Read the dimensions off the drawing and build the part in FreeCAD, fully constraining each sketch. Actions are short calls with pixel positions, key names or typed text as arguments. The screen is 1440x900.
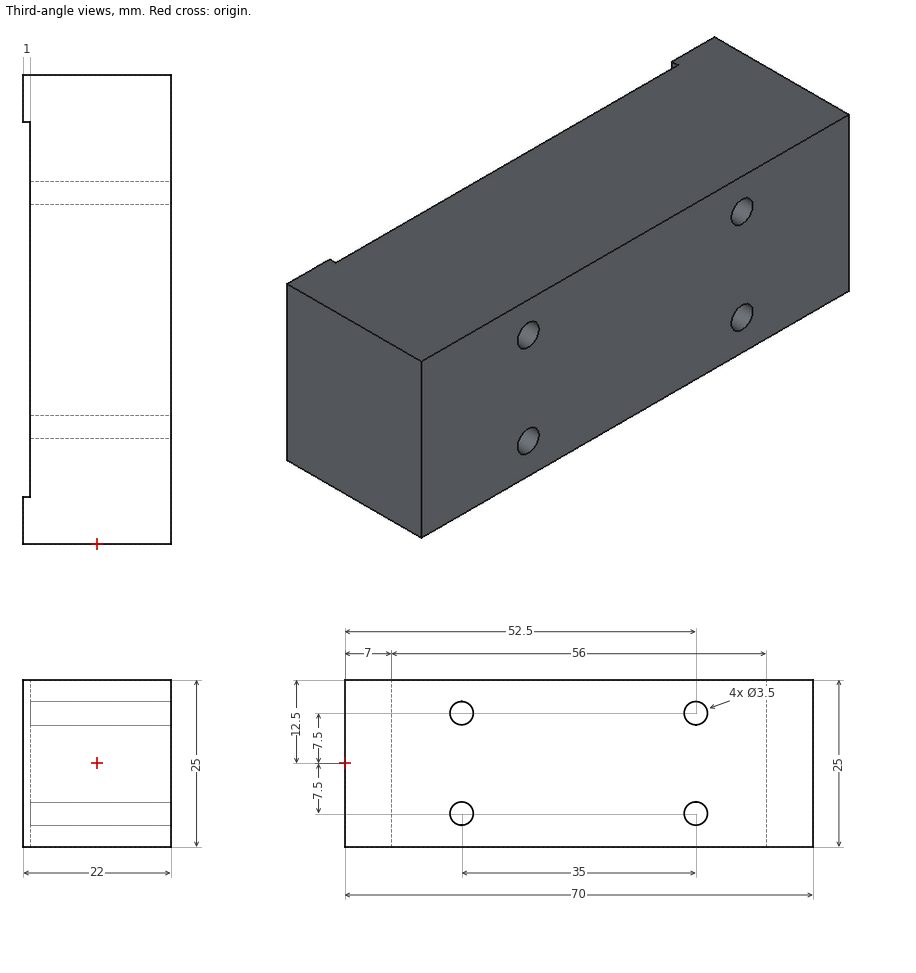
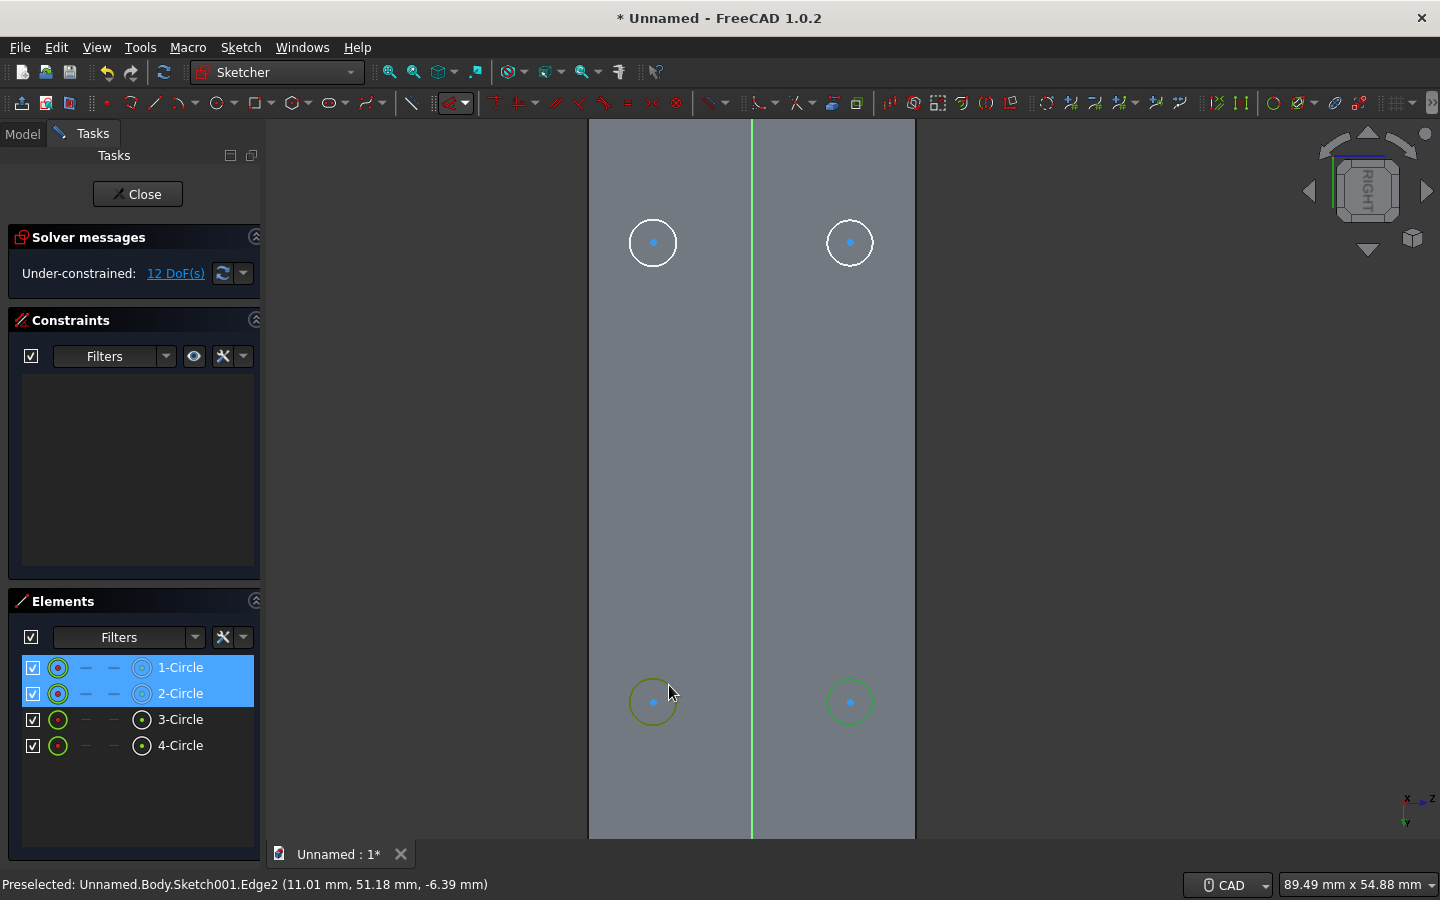
click(669, 226)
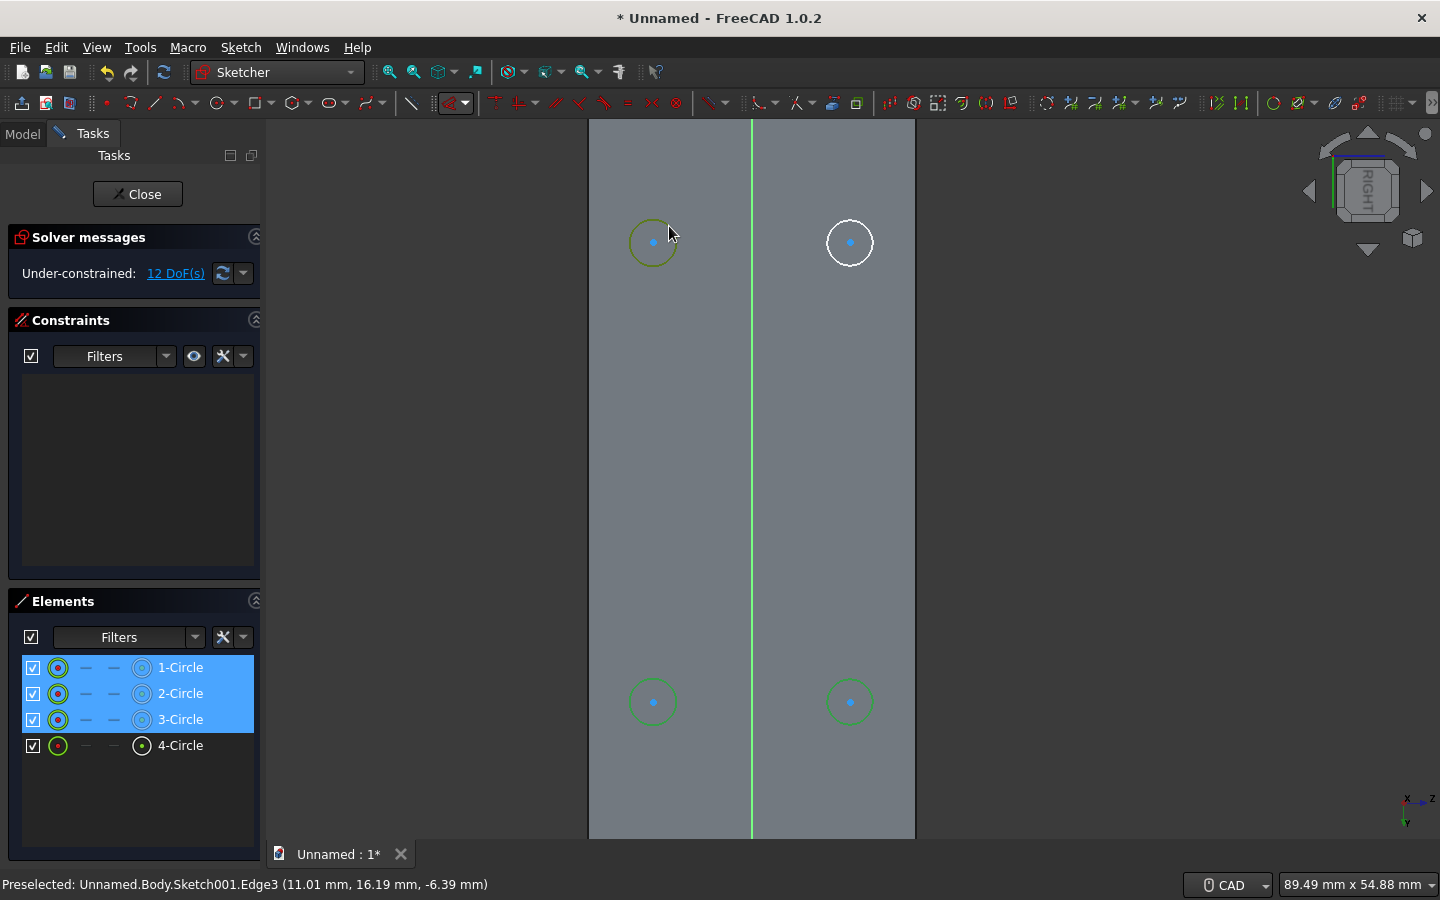
click(866, 227)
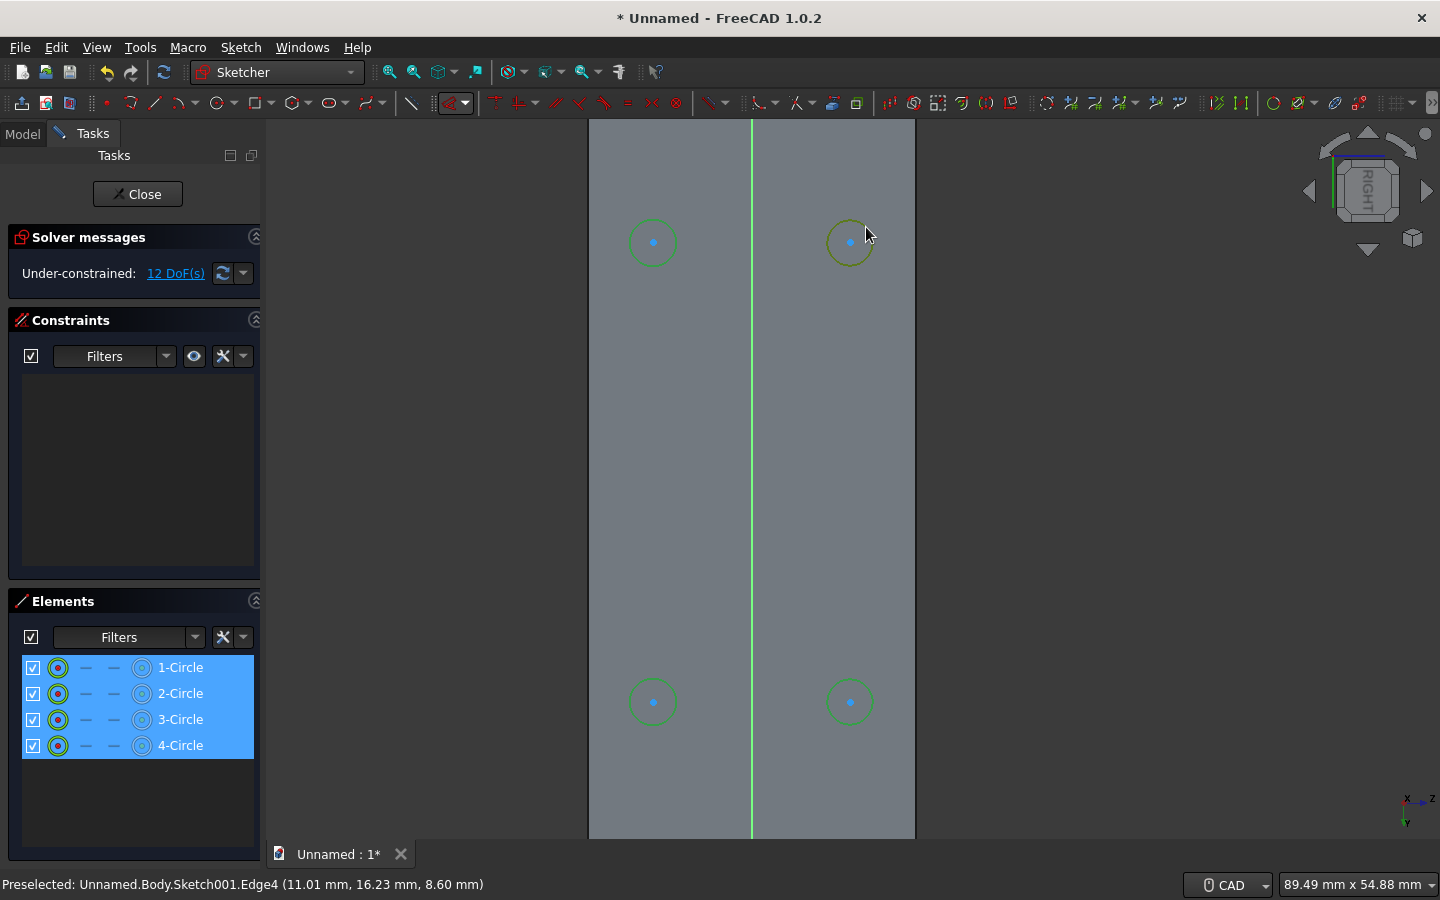
click(628, 104)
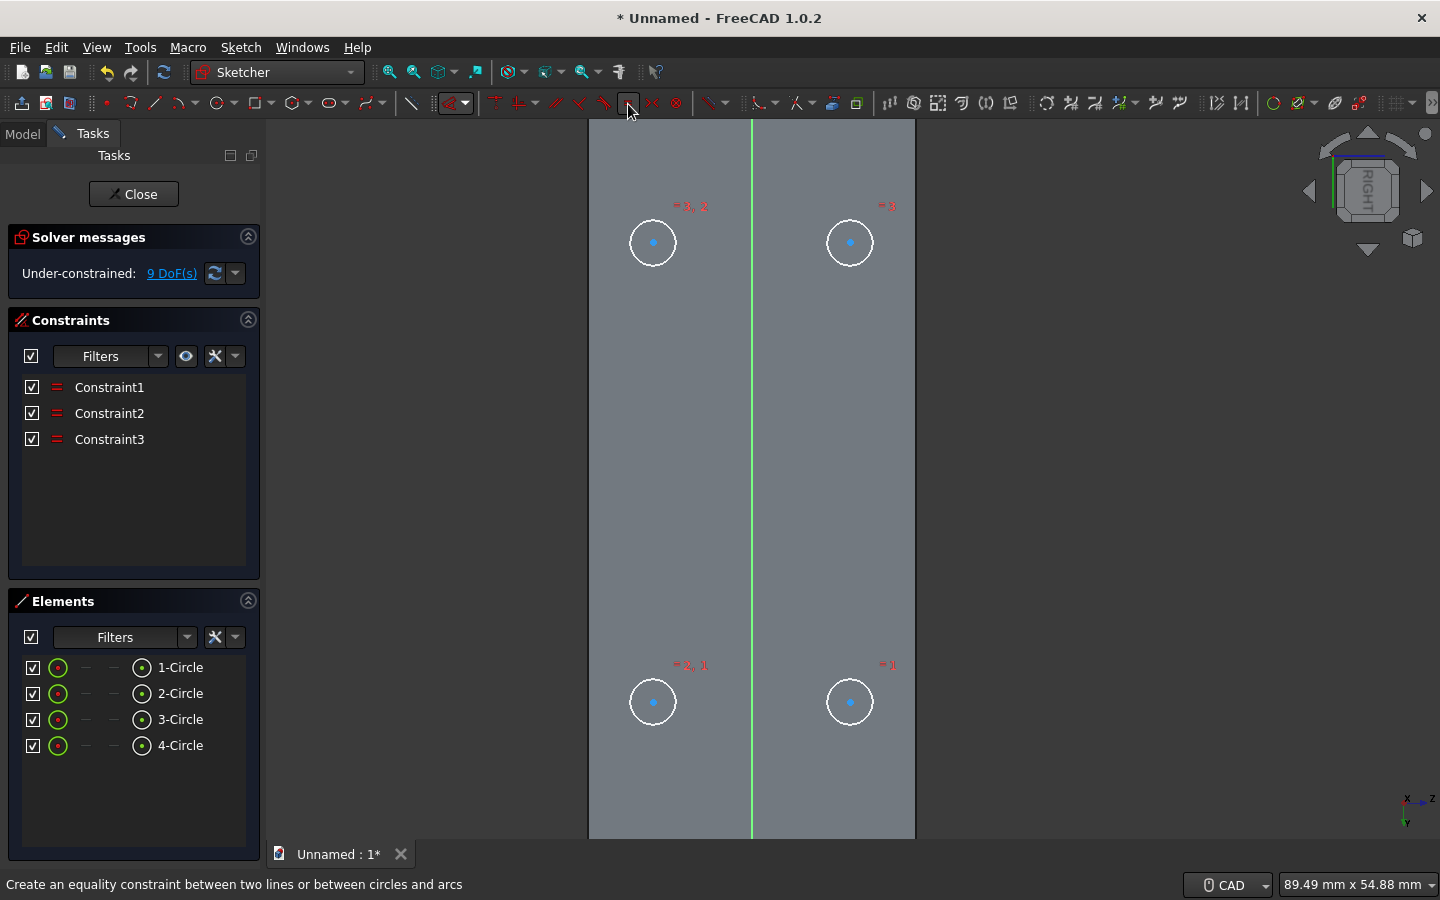
click(850, 702)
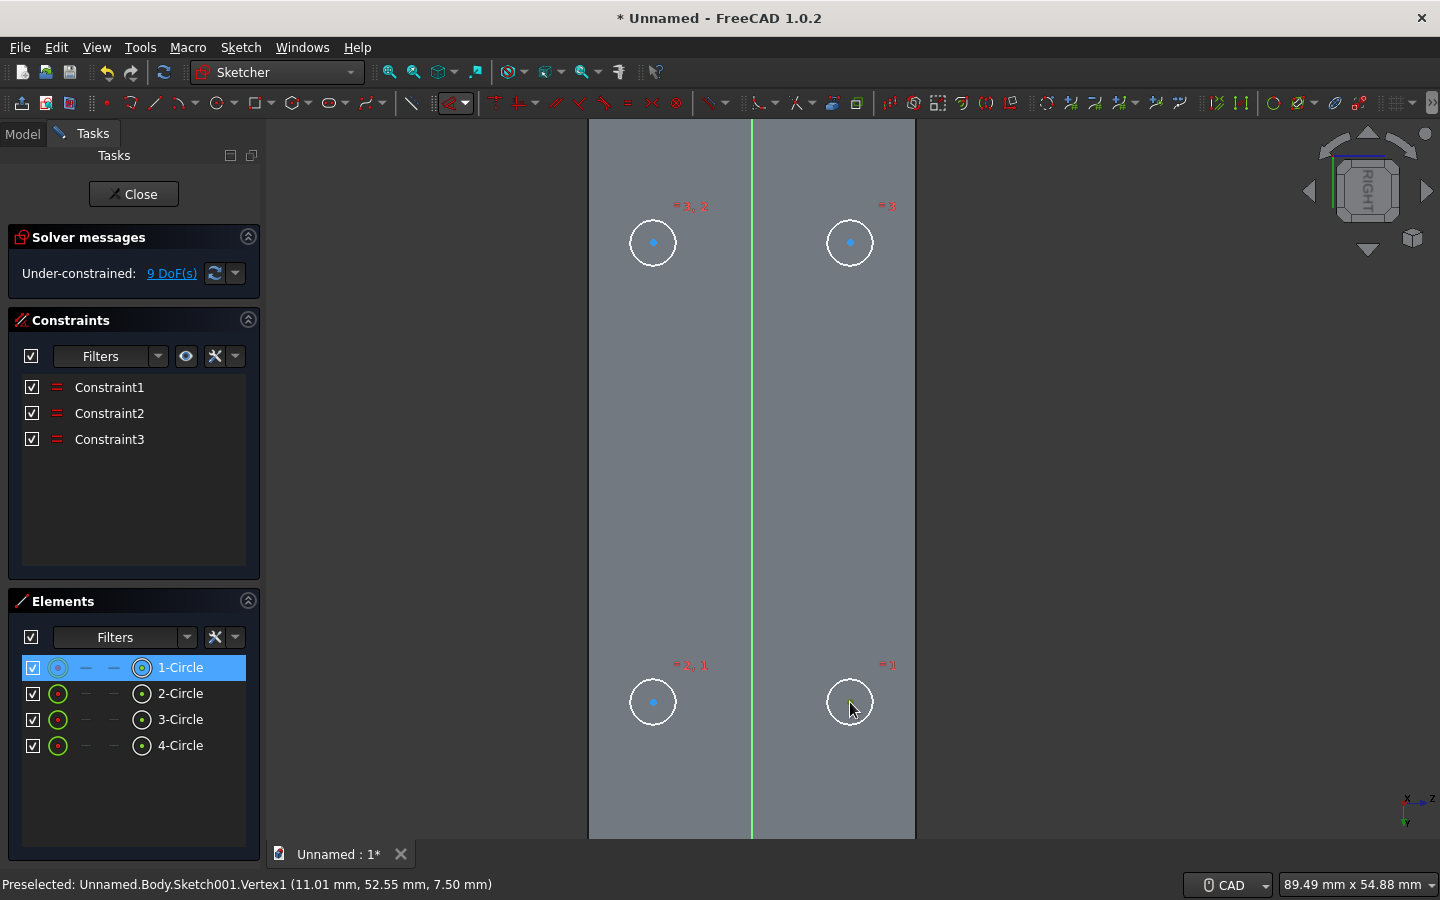
click(653, 702)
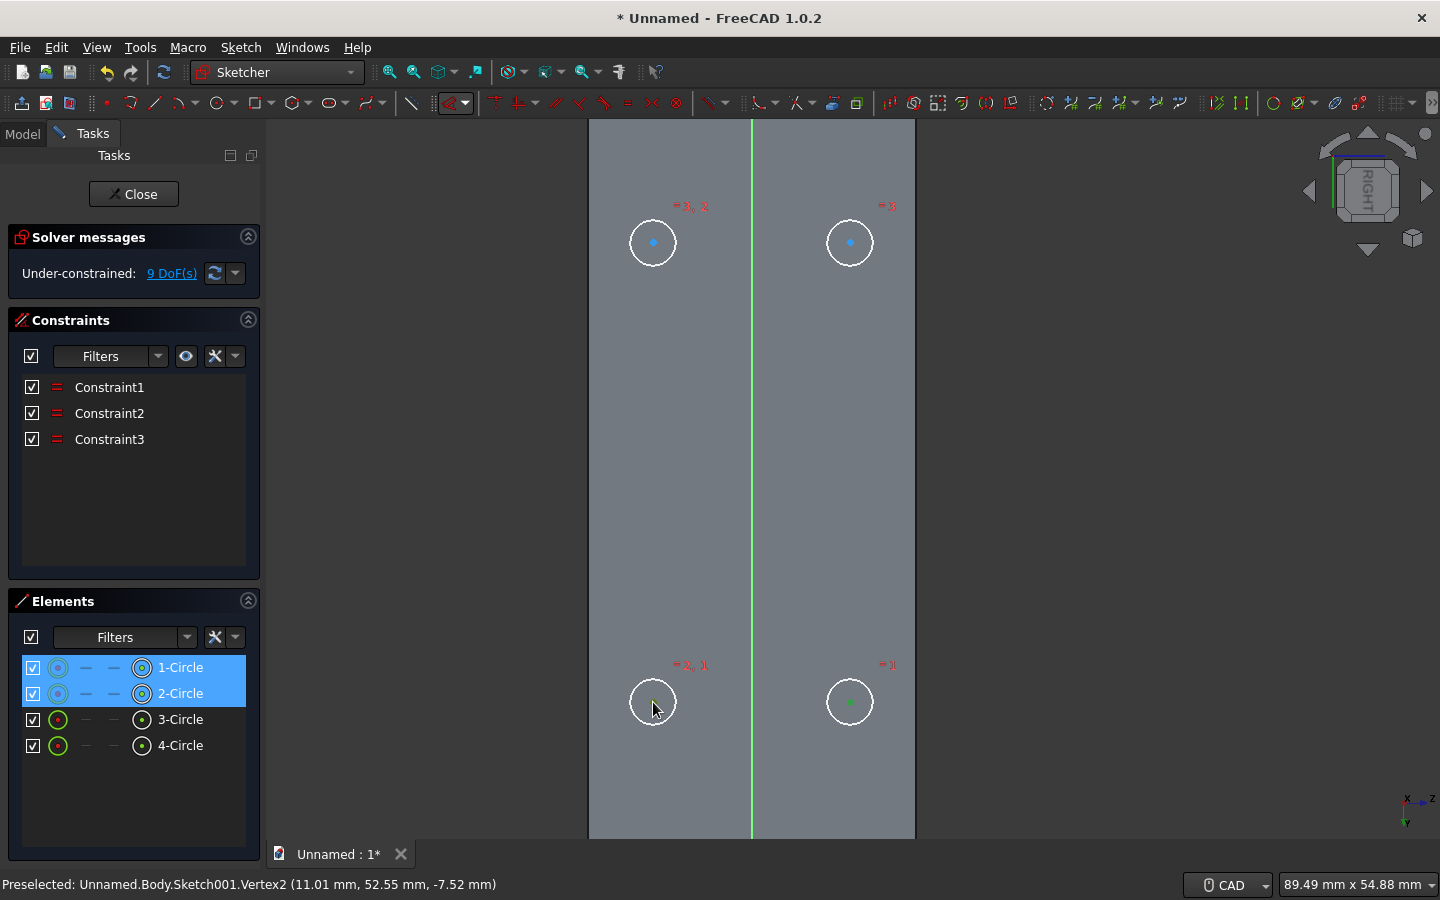
key(h)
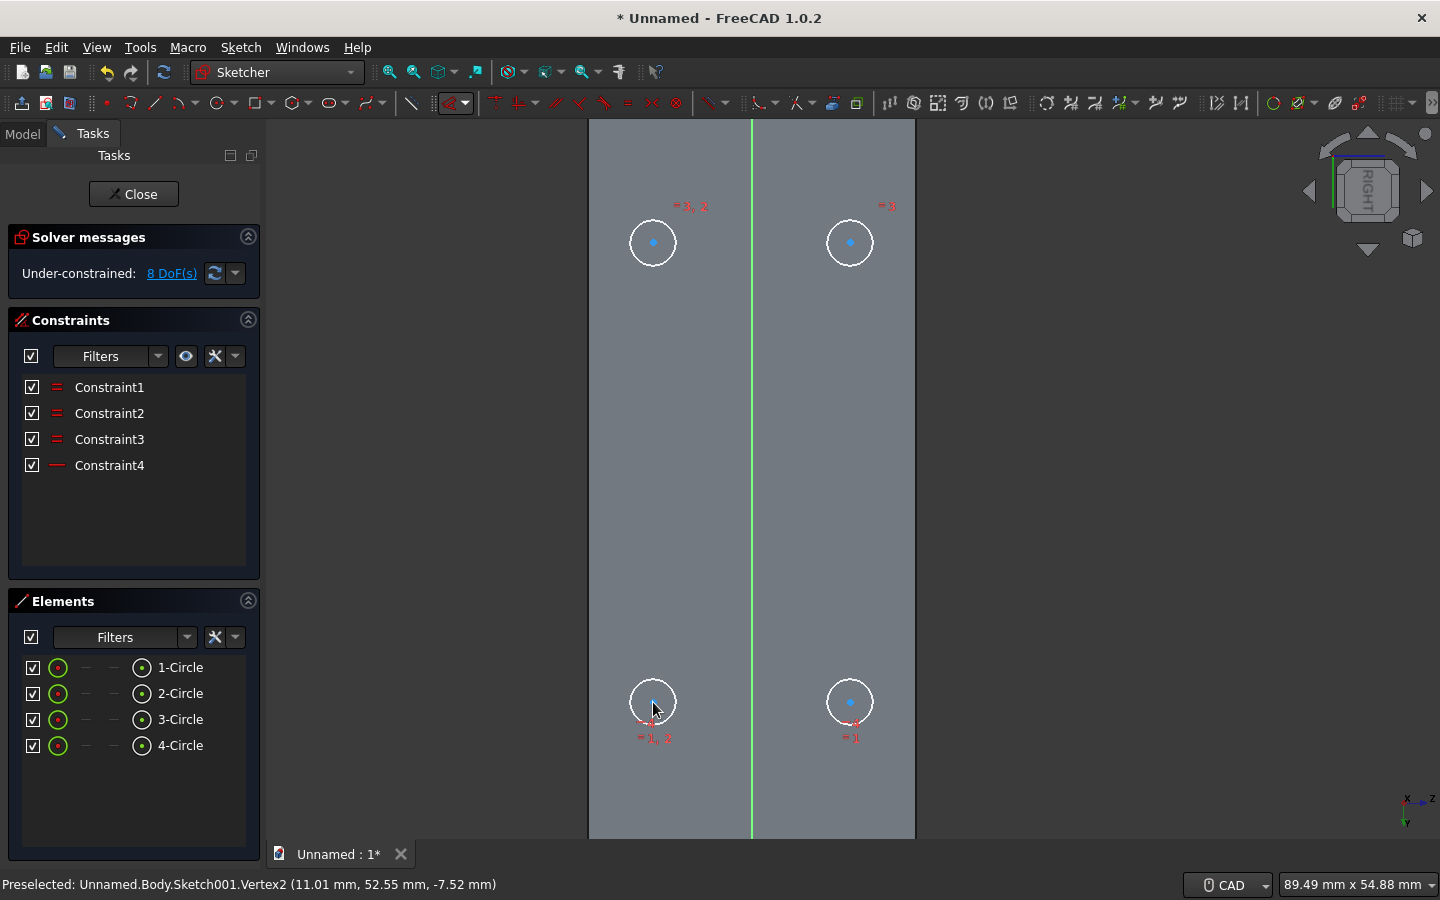
click(653, 702)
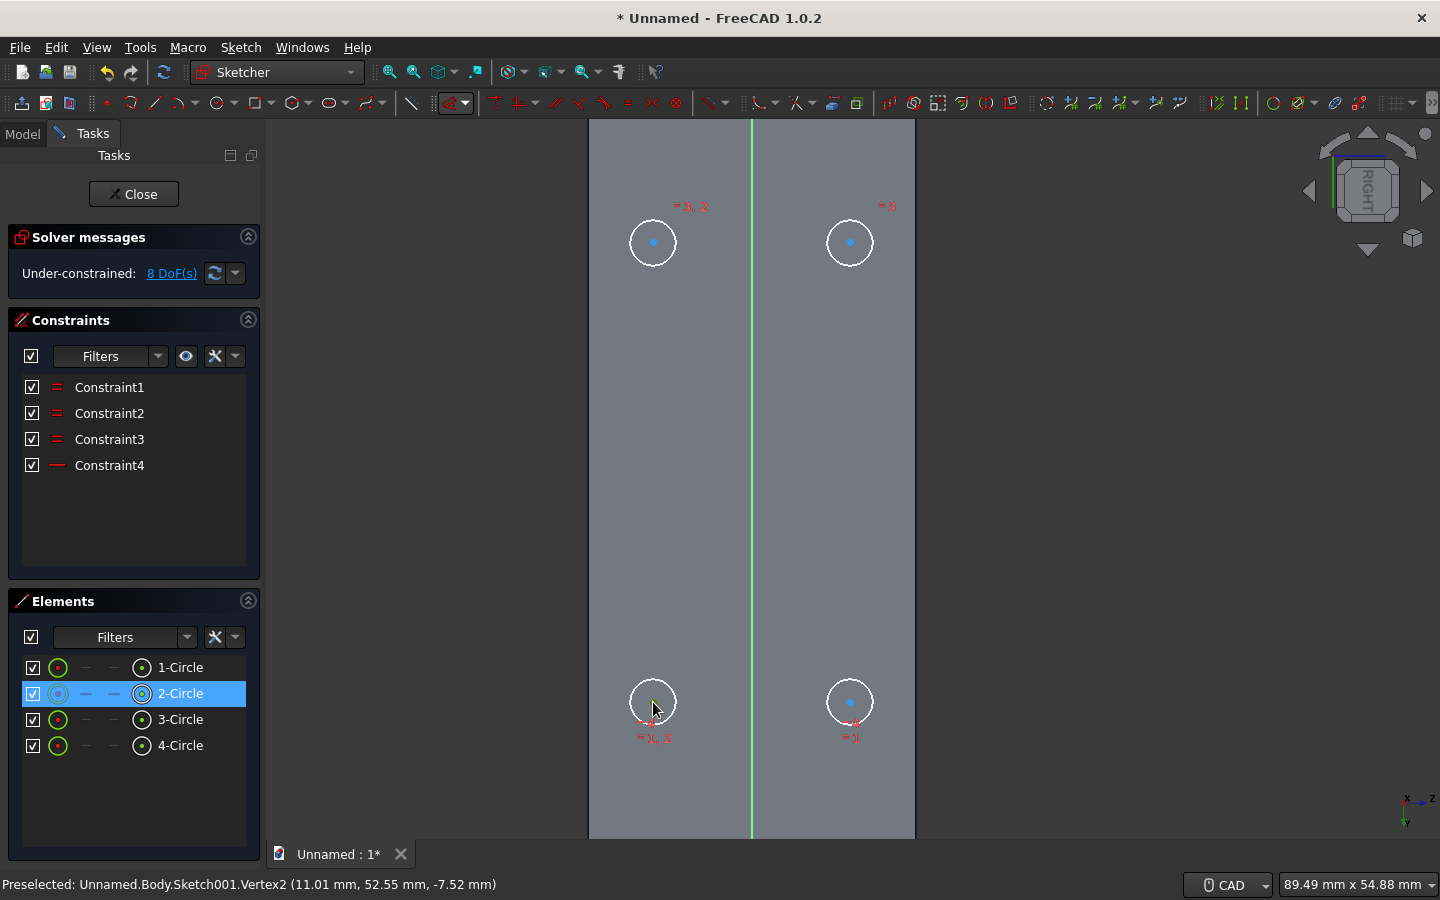
click(653, 243)